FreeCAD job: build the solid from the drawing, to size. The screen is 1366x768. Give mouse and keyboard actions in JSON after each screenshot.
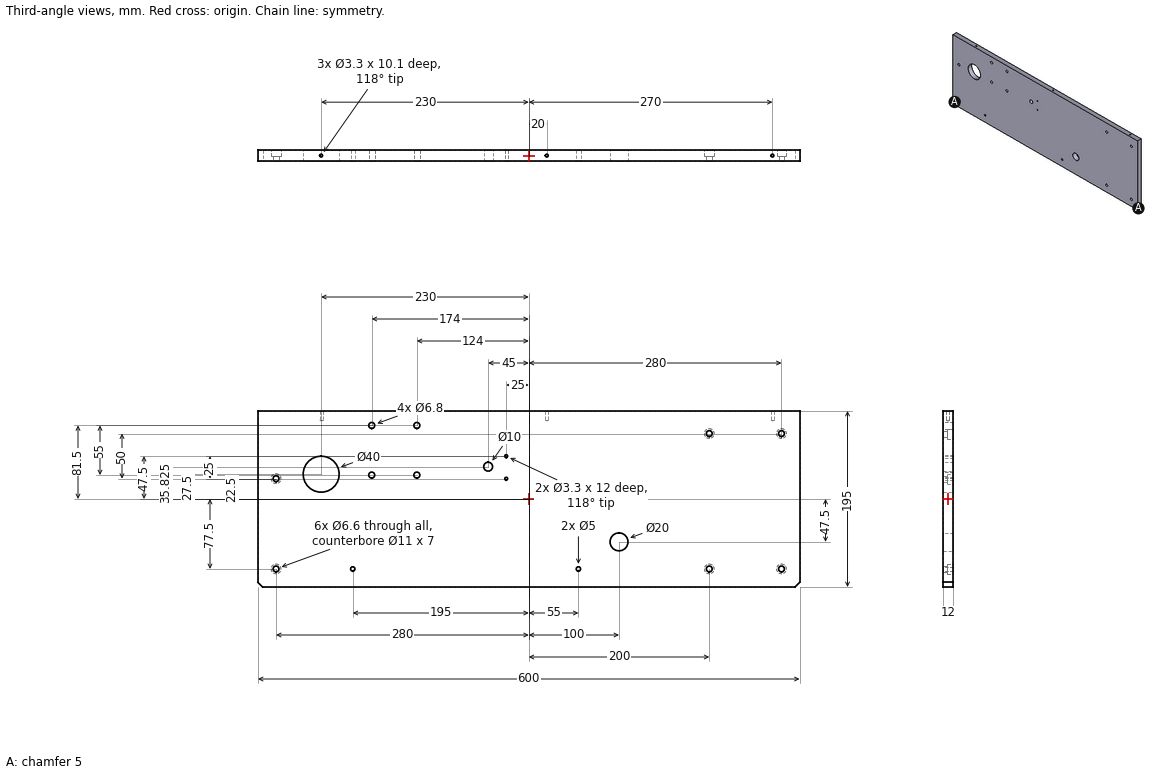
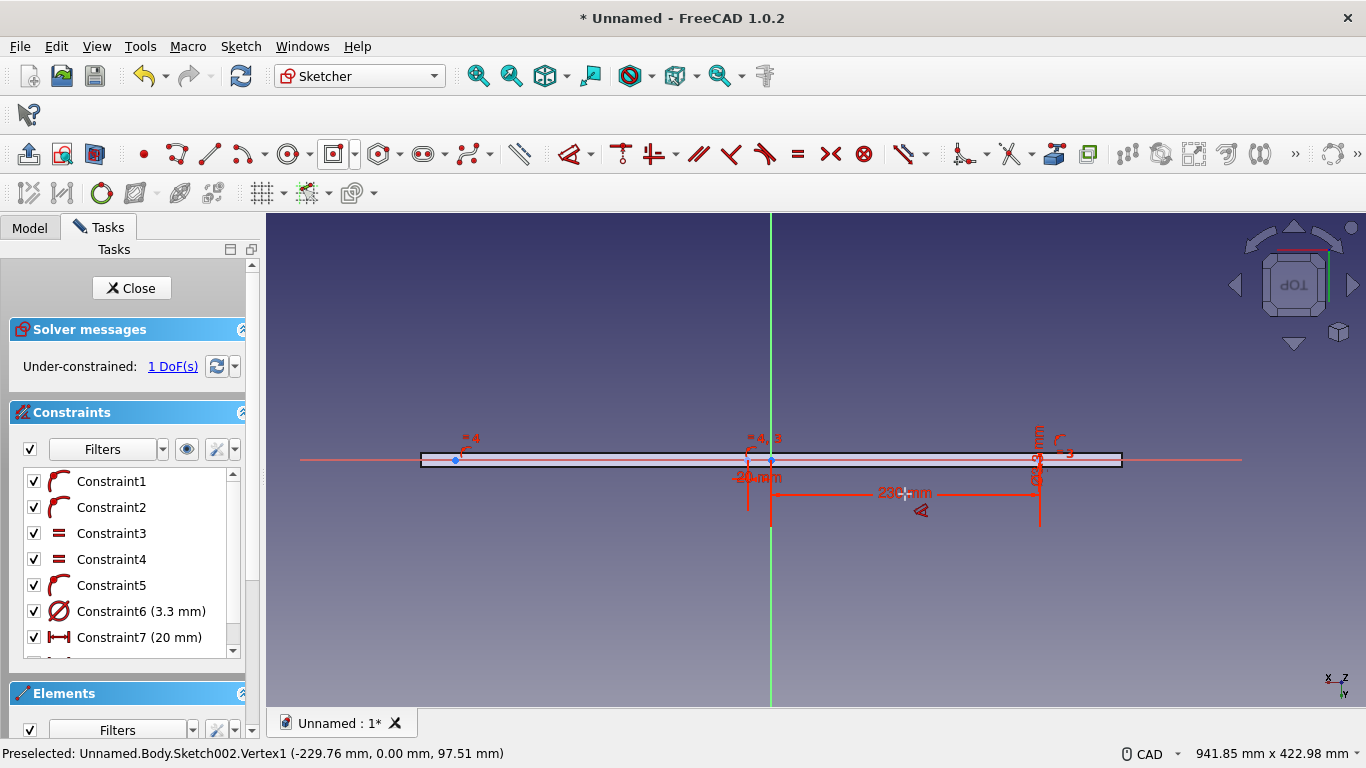
{"action": "left_click", "coordinate": [455, 460]}
{"action": "left_click", "coordinate": [613, 494]}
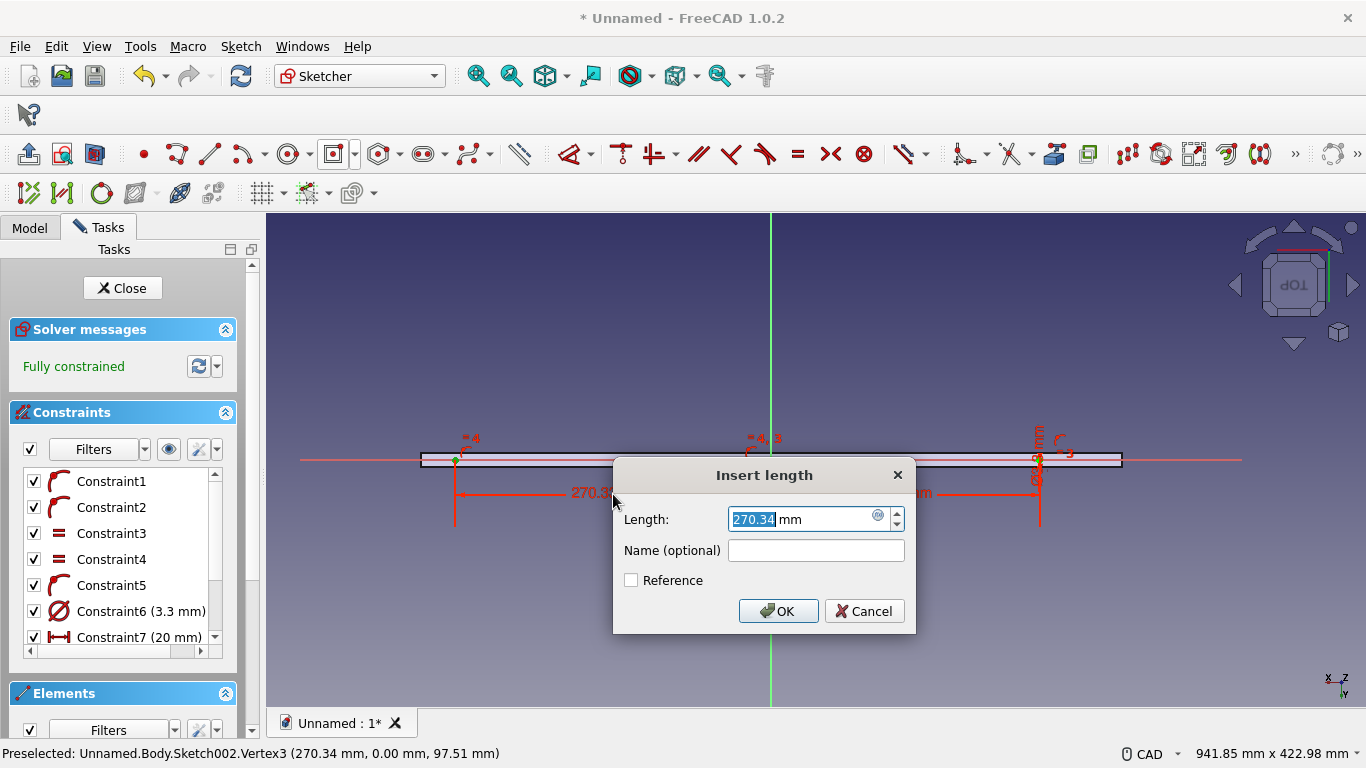
{"action": "type", "text": "270"}
{"action": "key", "text": "Return"}
{"action": "key", "text": "Escape"}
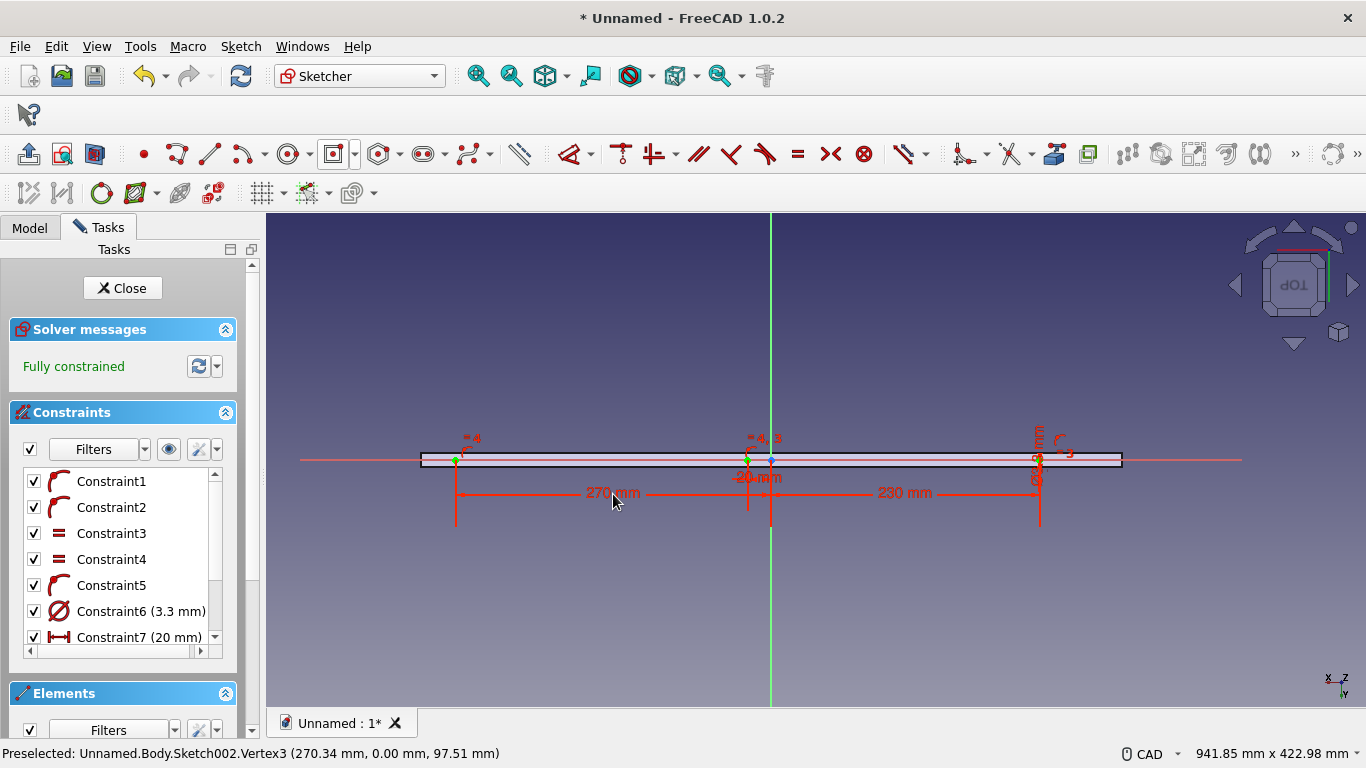
{"action": "left_click", "coordinate": [123, 288]}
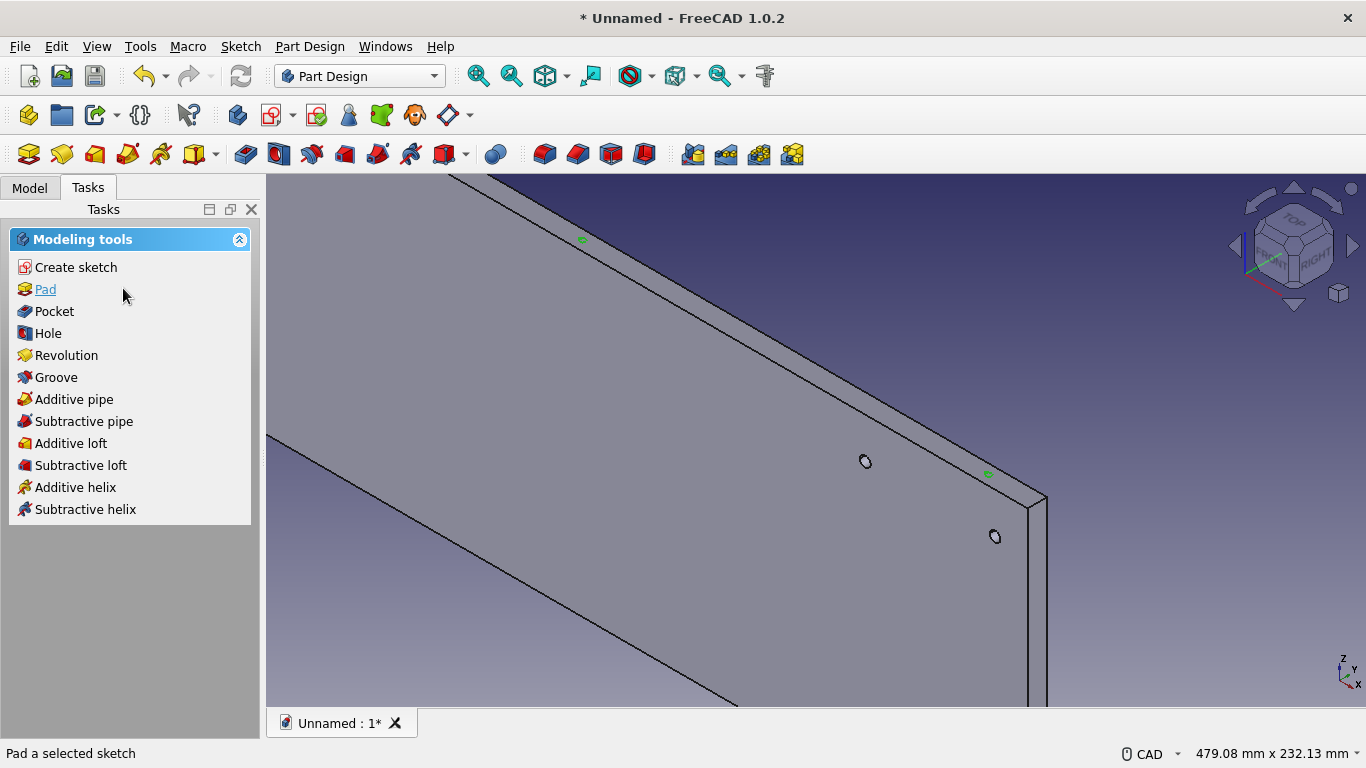
{"action": "left_click", "coordinate": [279, 154]}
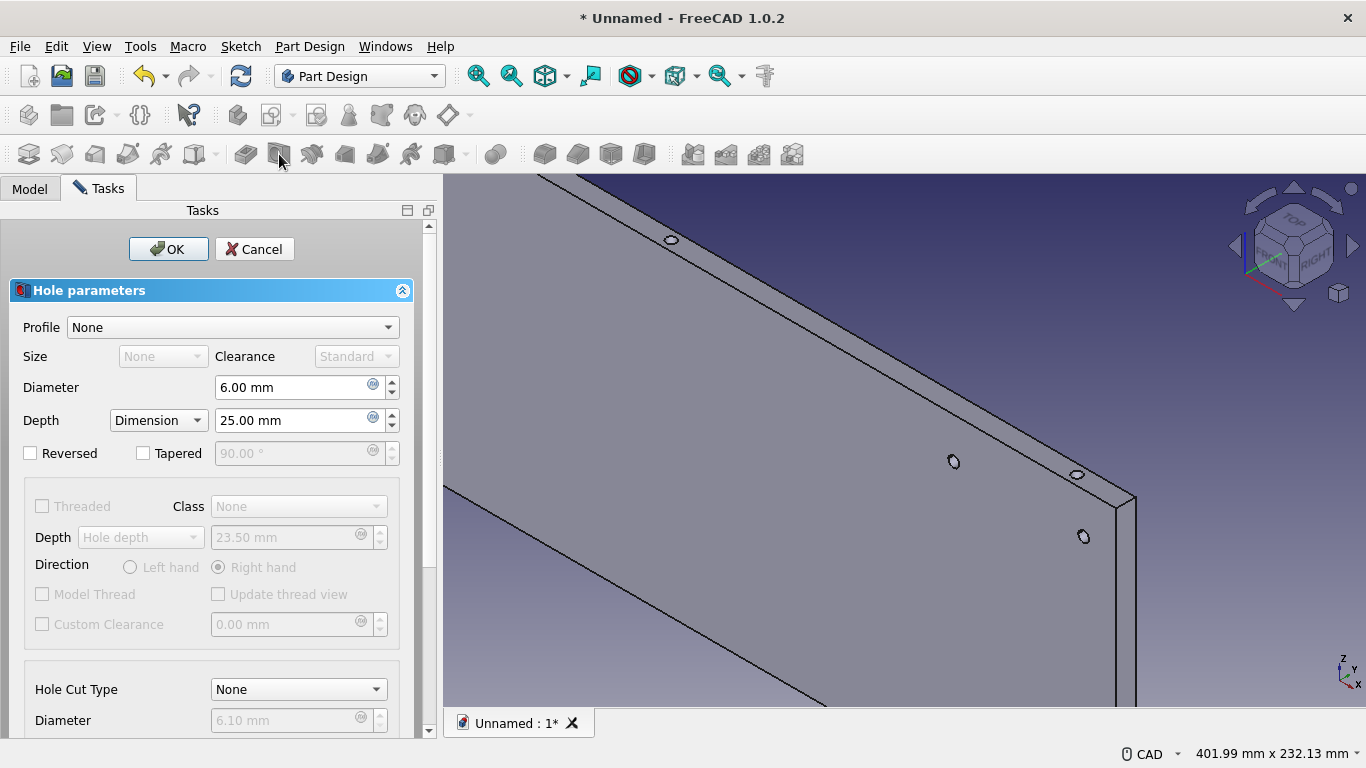
{"action": "triple_click", "coordinate": [300, 388]}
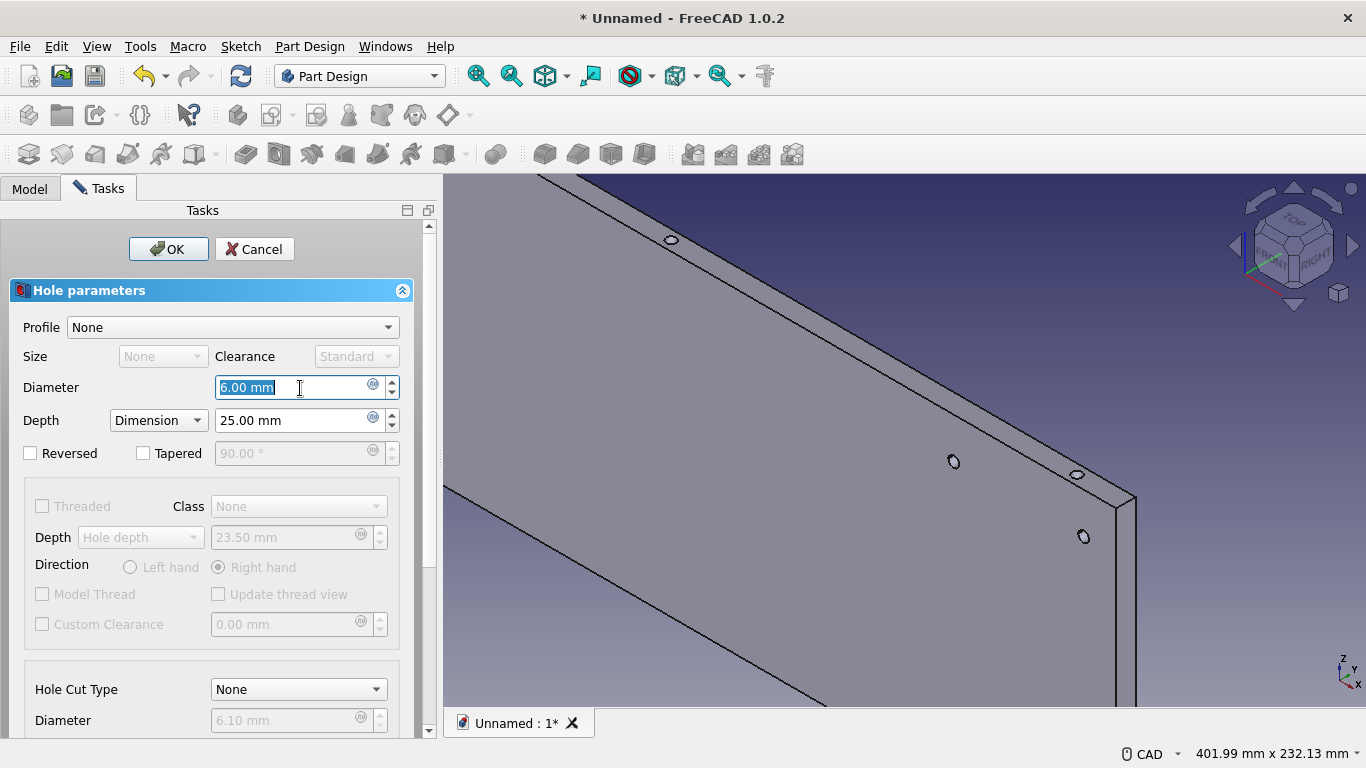
{"action": "type", "text": "3.3"}
{"action": "key", "text": "Tab"}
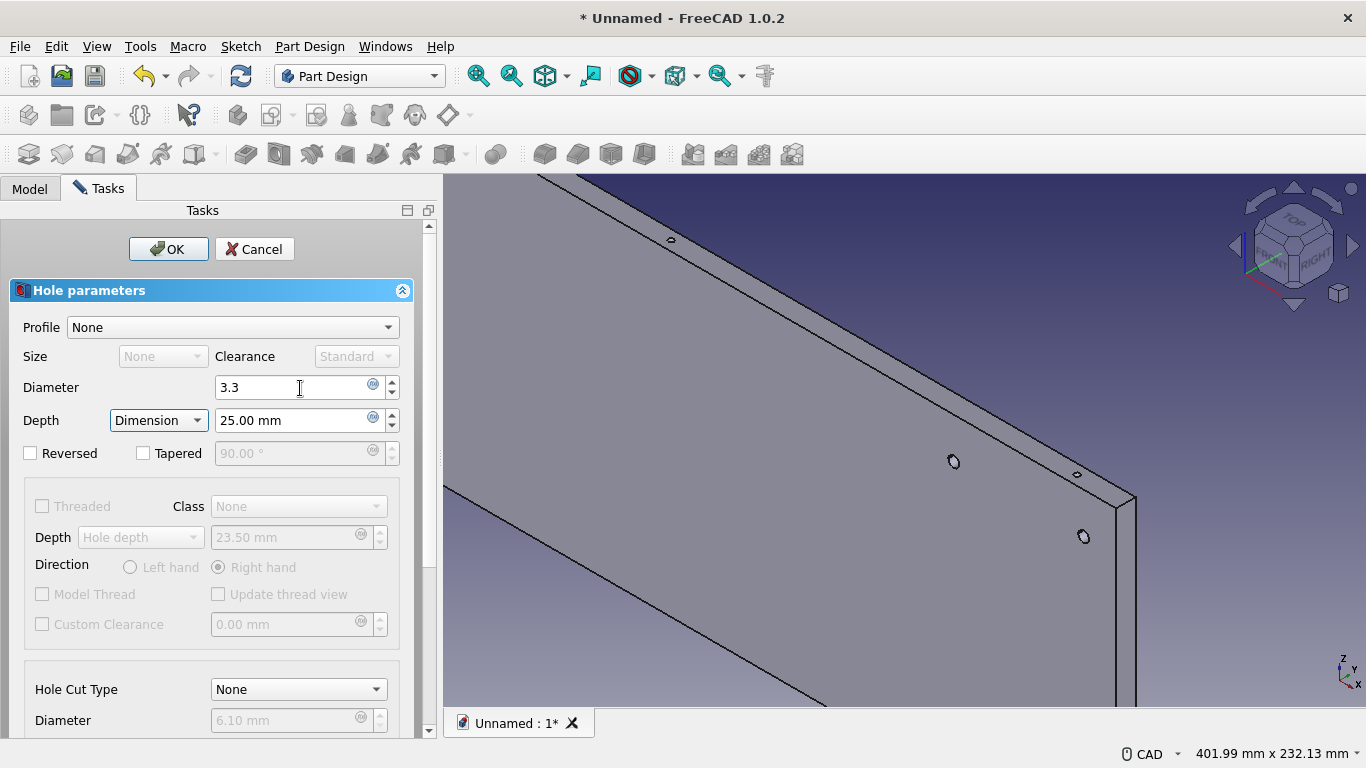
{"action": "triple_click", "coordinate": [300, 420]}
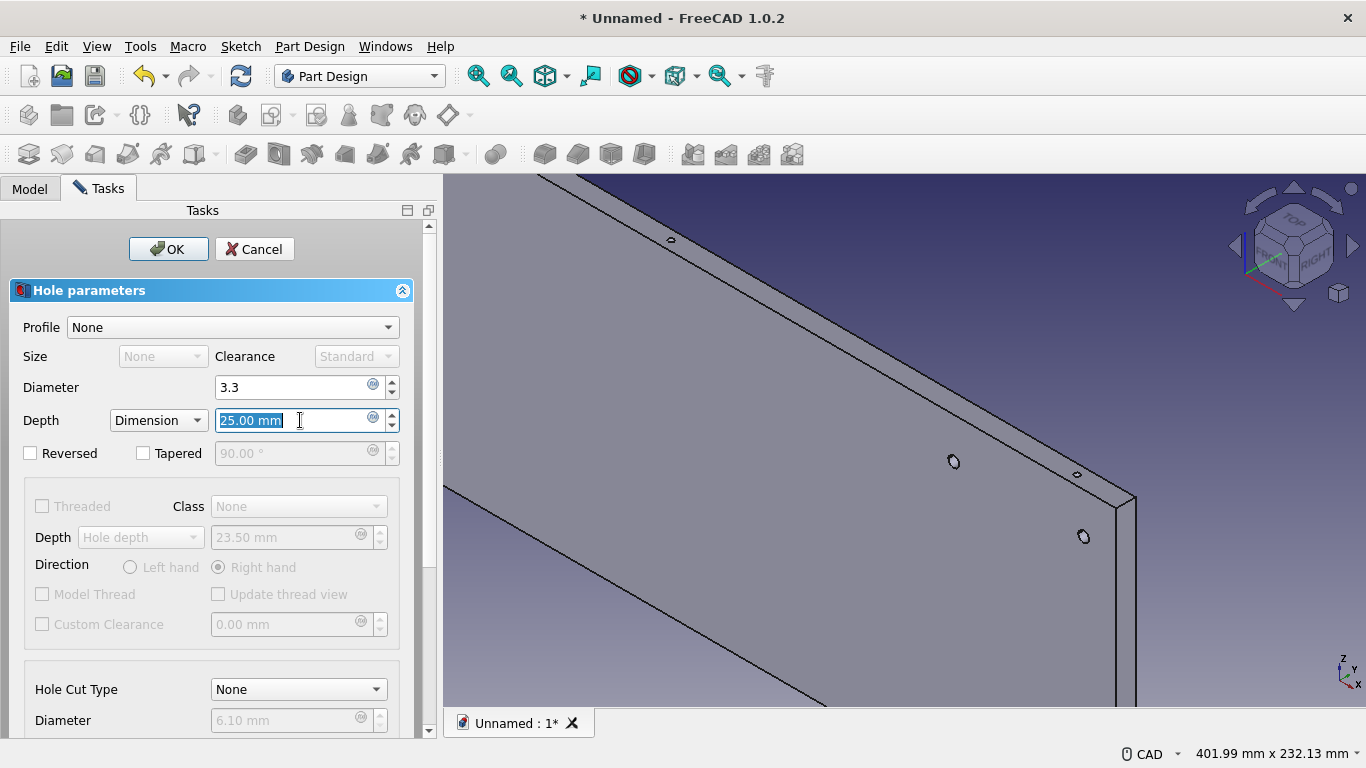
{"action": "type", "text": "10.1"}
{"action": "key", "text": "Tab"}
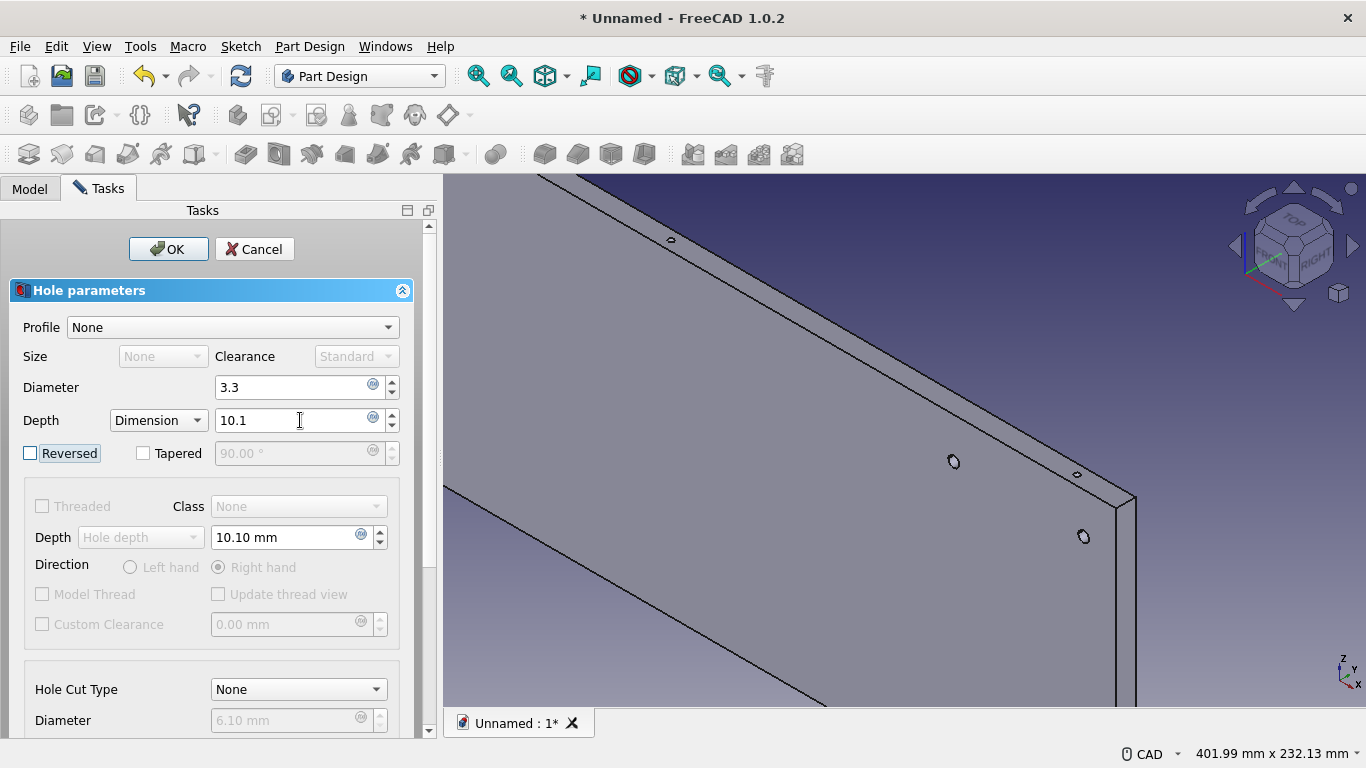
{"action": "left_click", "coordinate": [169, 249]}